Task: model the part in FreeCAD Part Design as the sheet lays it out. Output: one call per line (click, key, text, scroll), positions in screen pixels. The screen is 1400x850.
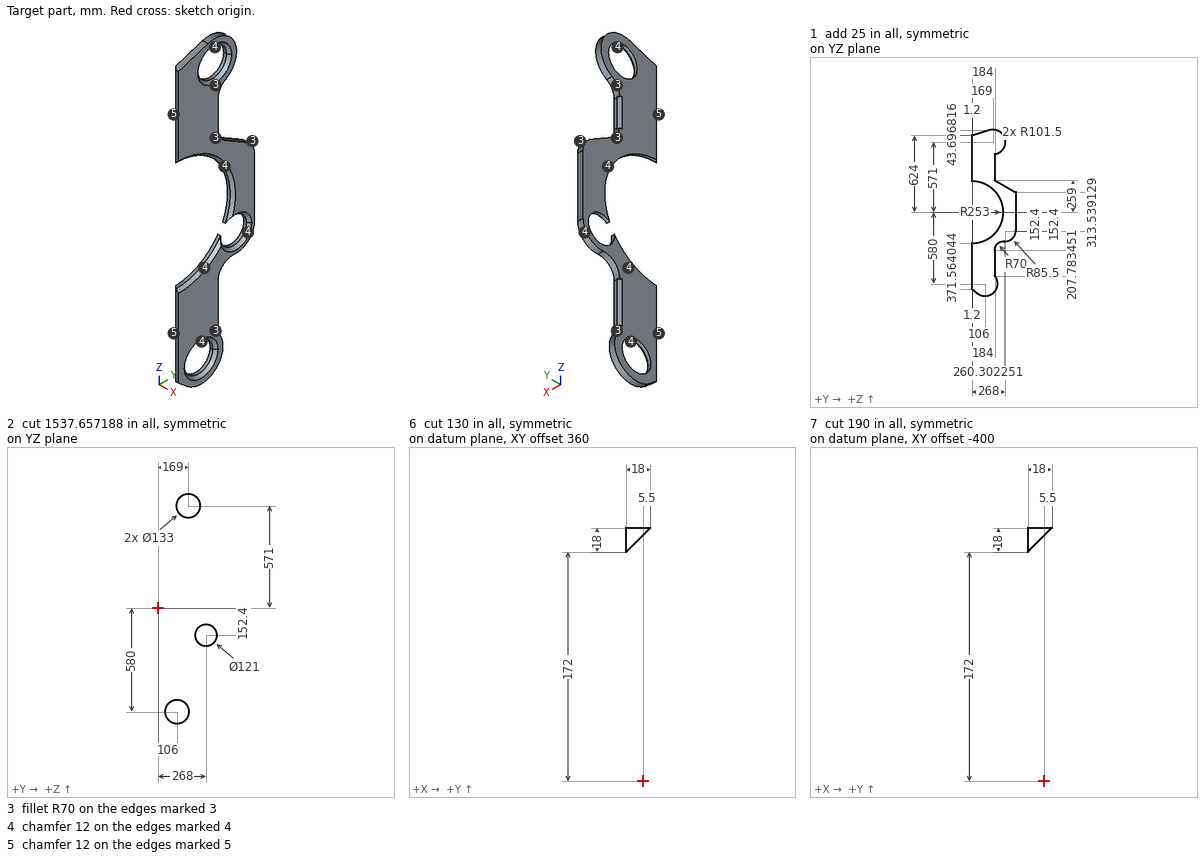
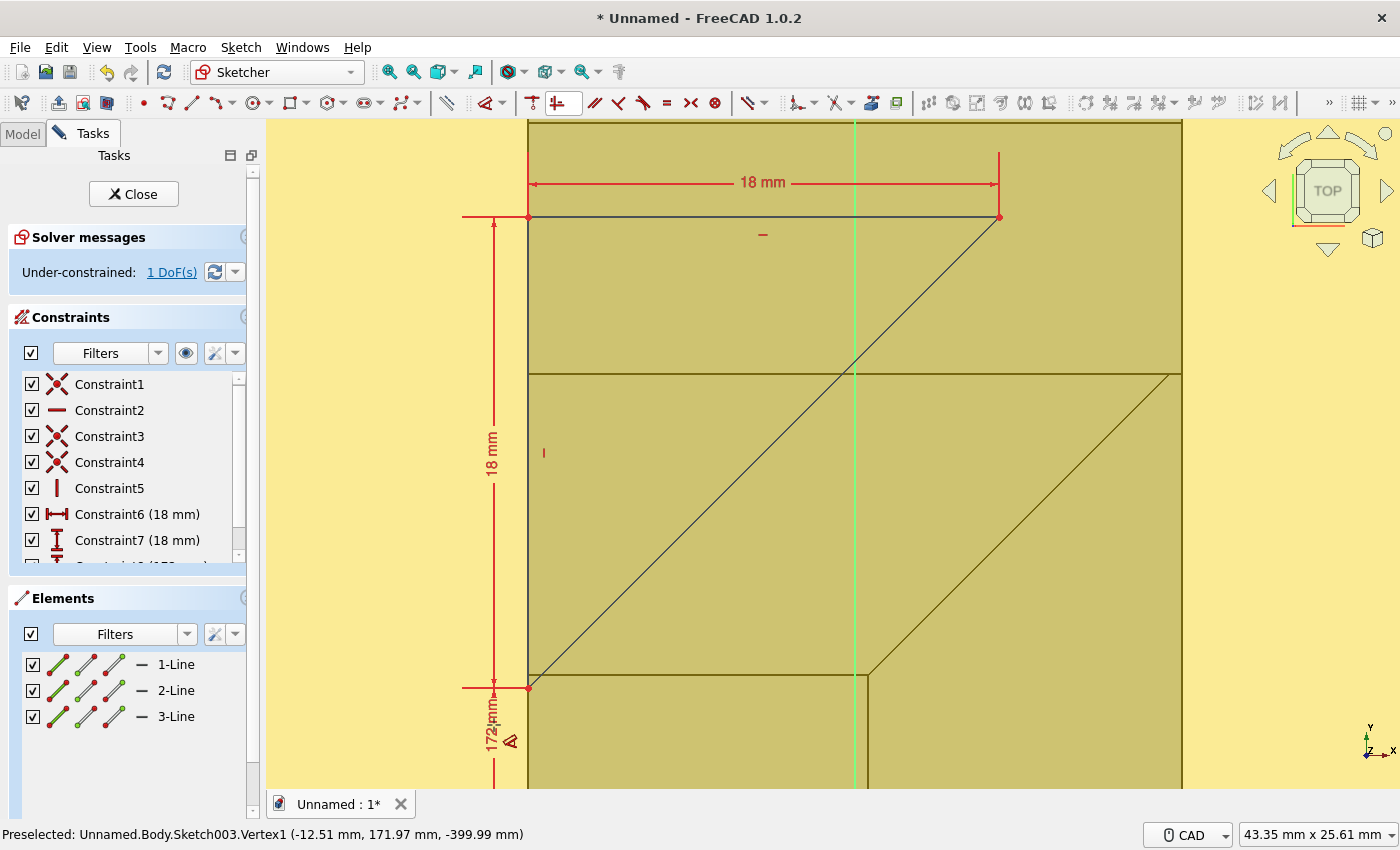
click(999, 217)
click(927, 183)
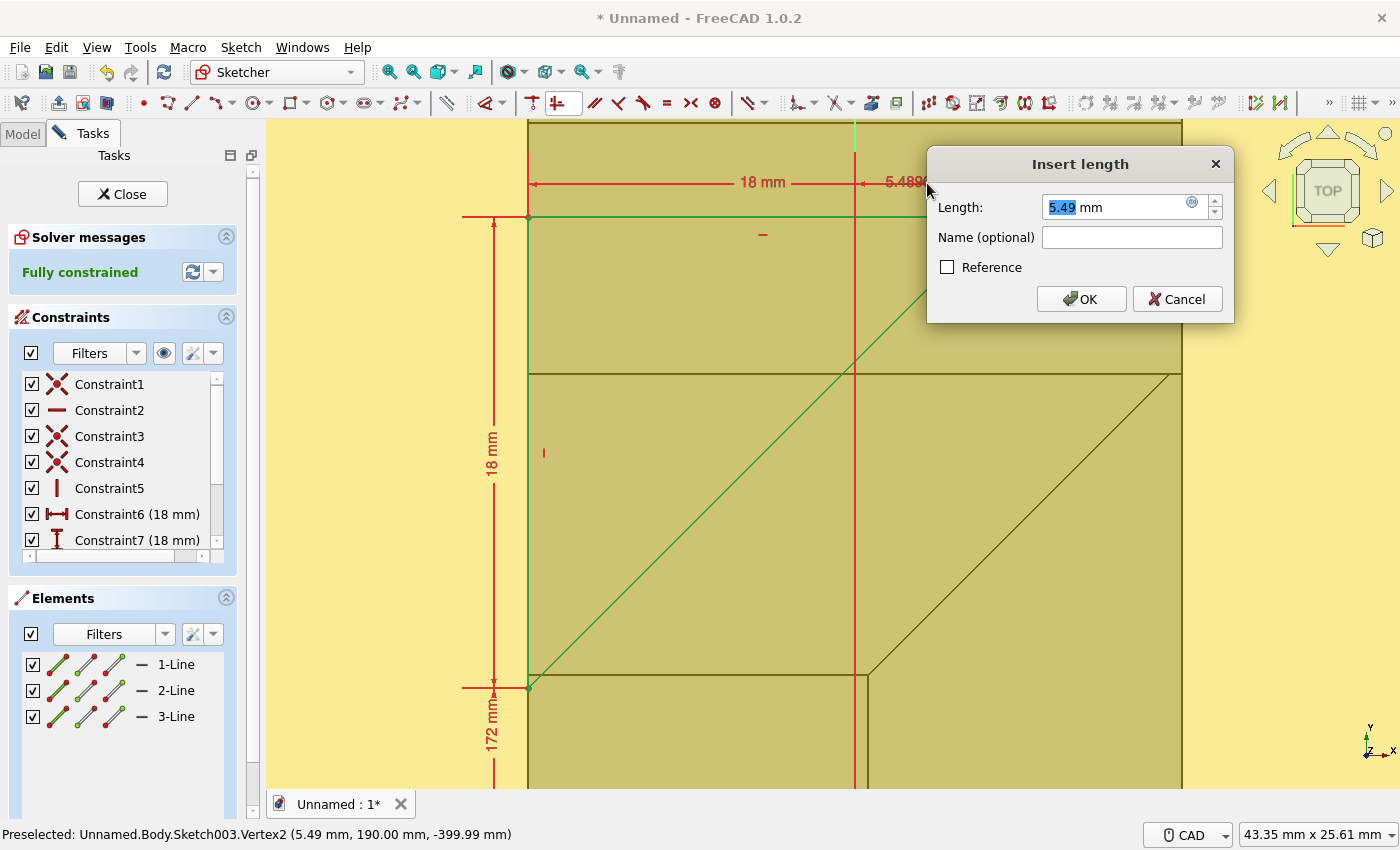
text(5.5)
key(Return)
key(Escape)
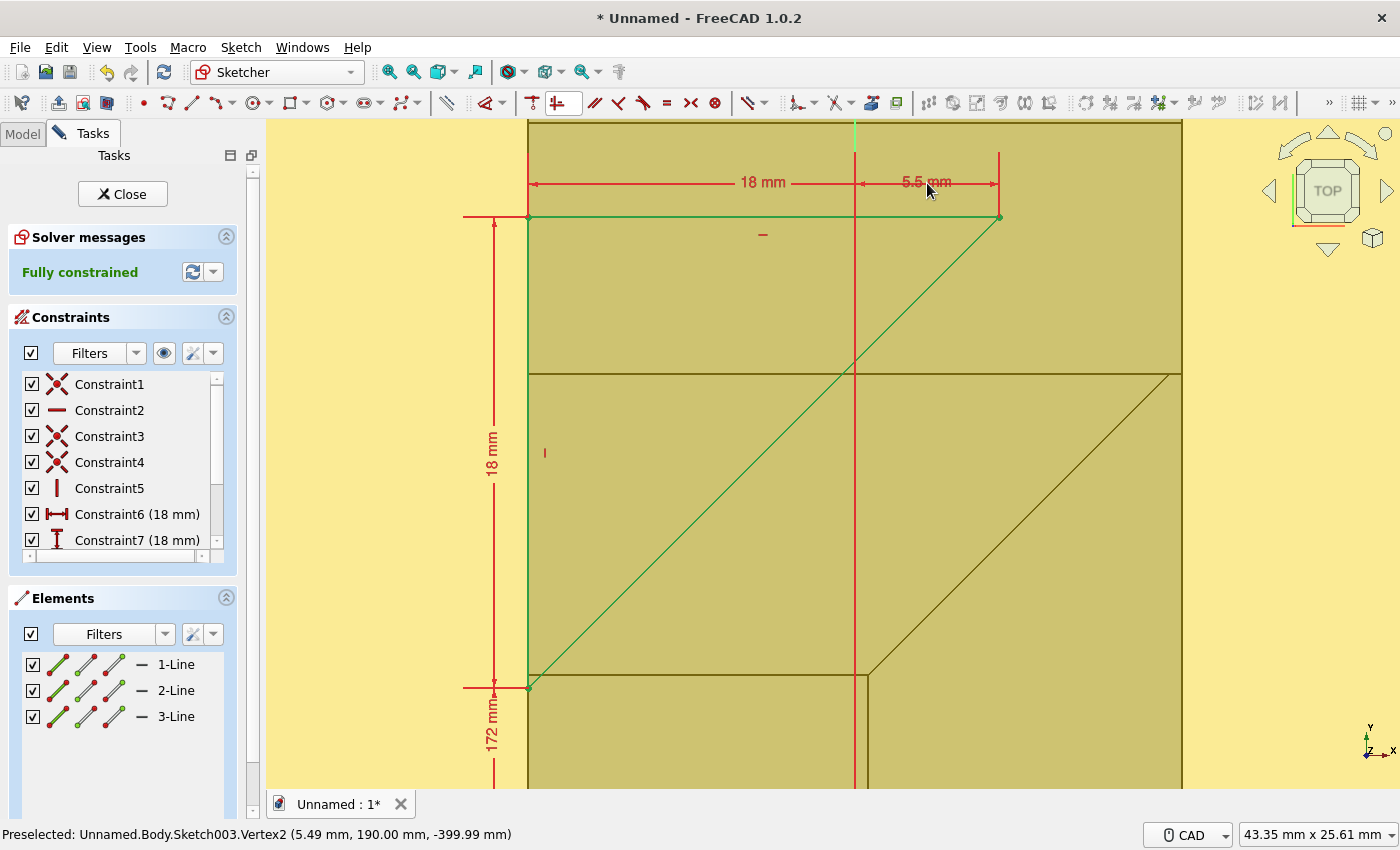
click(123, 194)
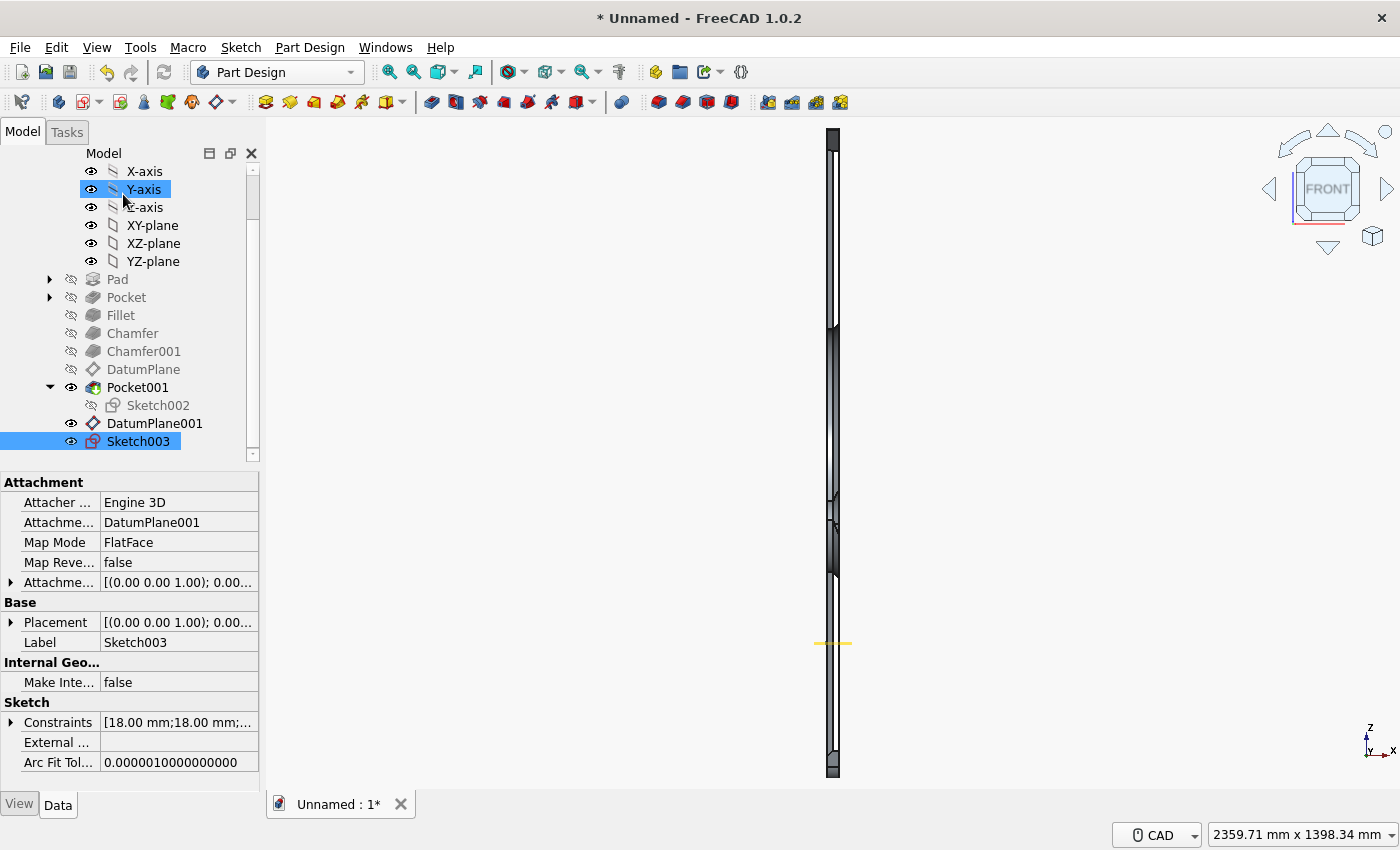
click(432, 102)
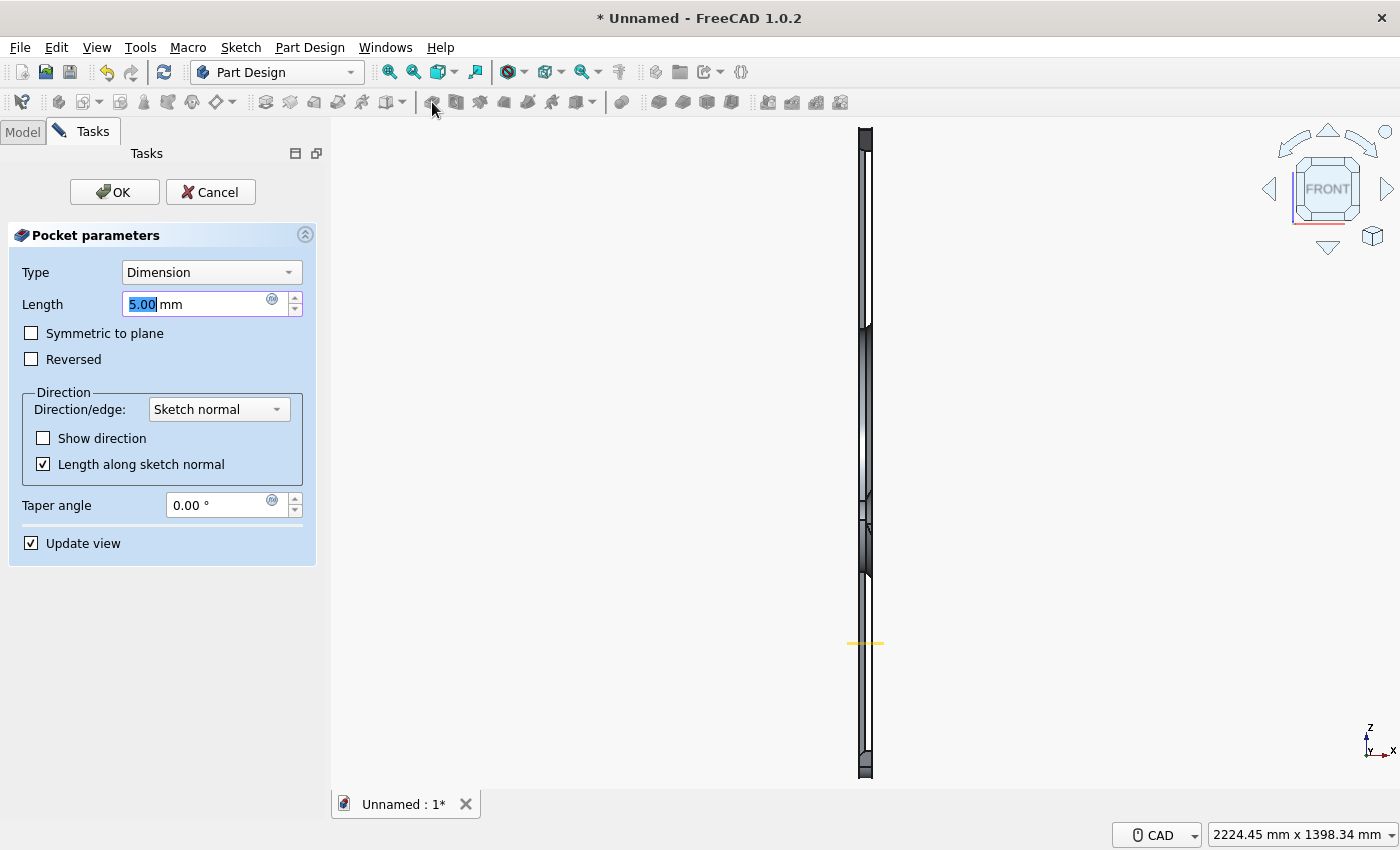
text(190)
key(Tab)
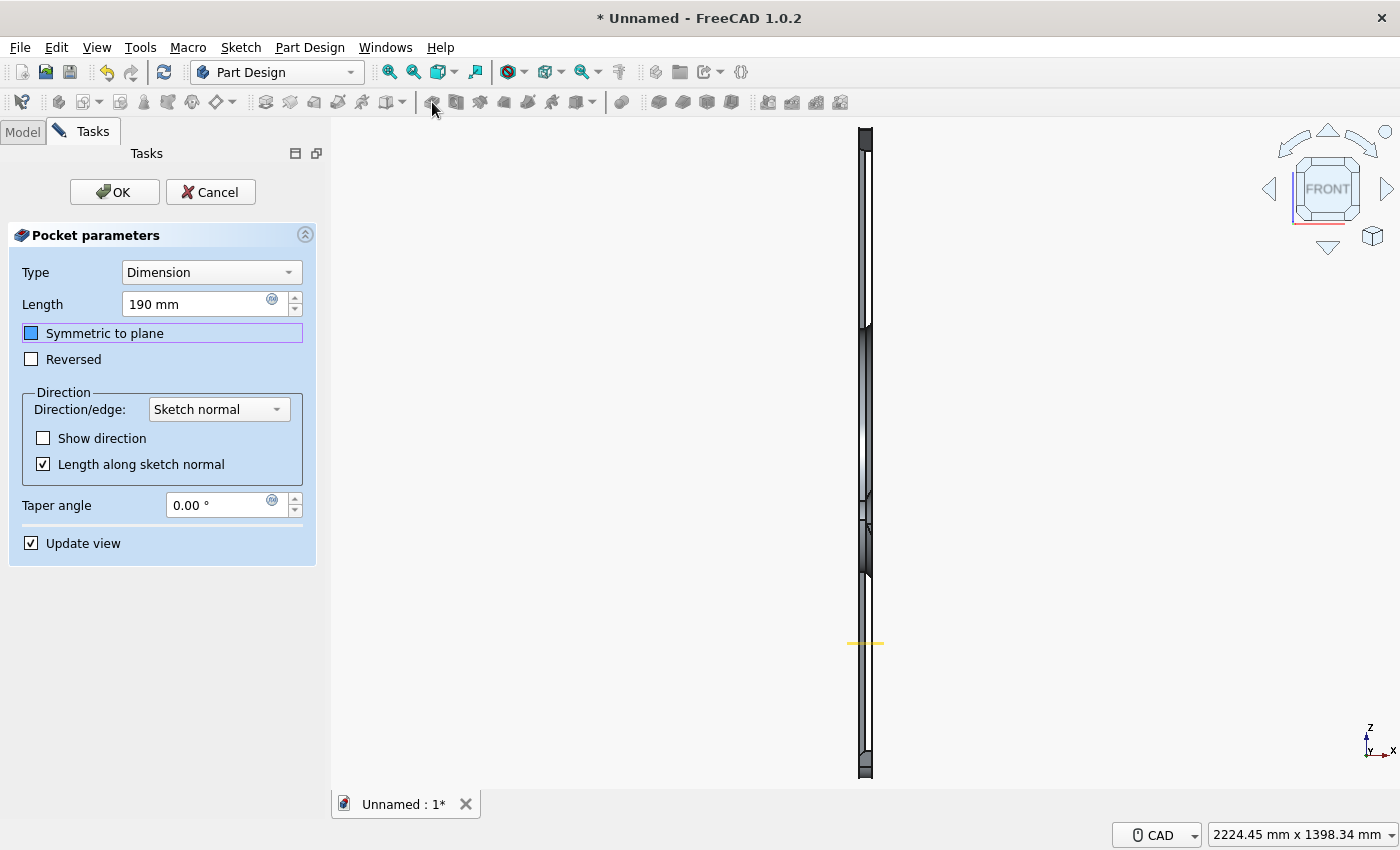
click(30, 333)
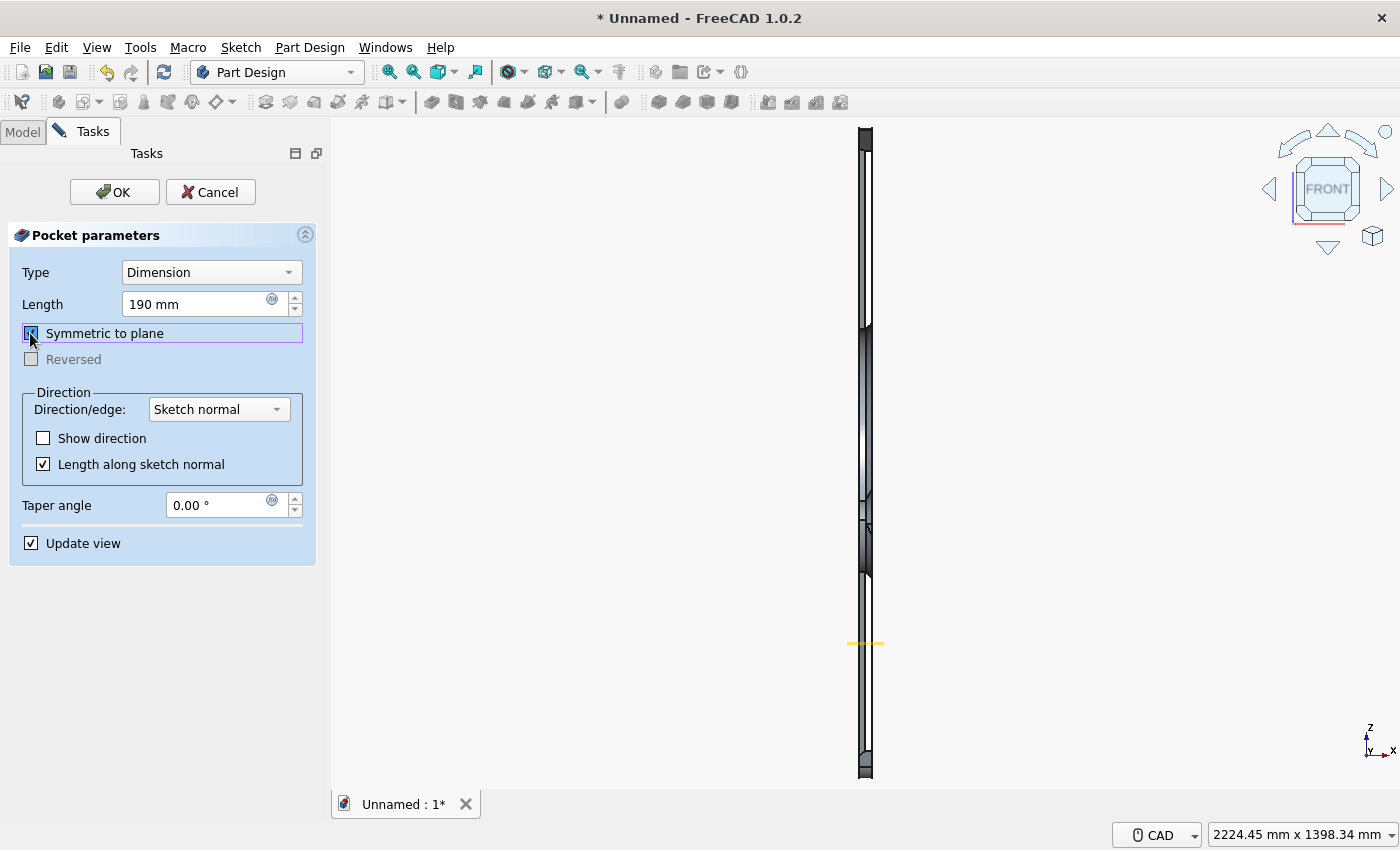
click(115, 192)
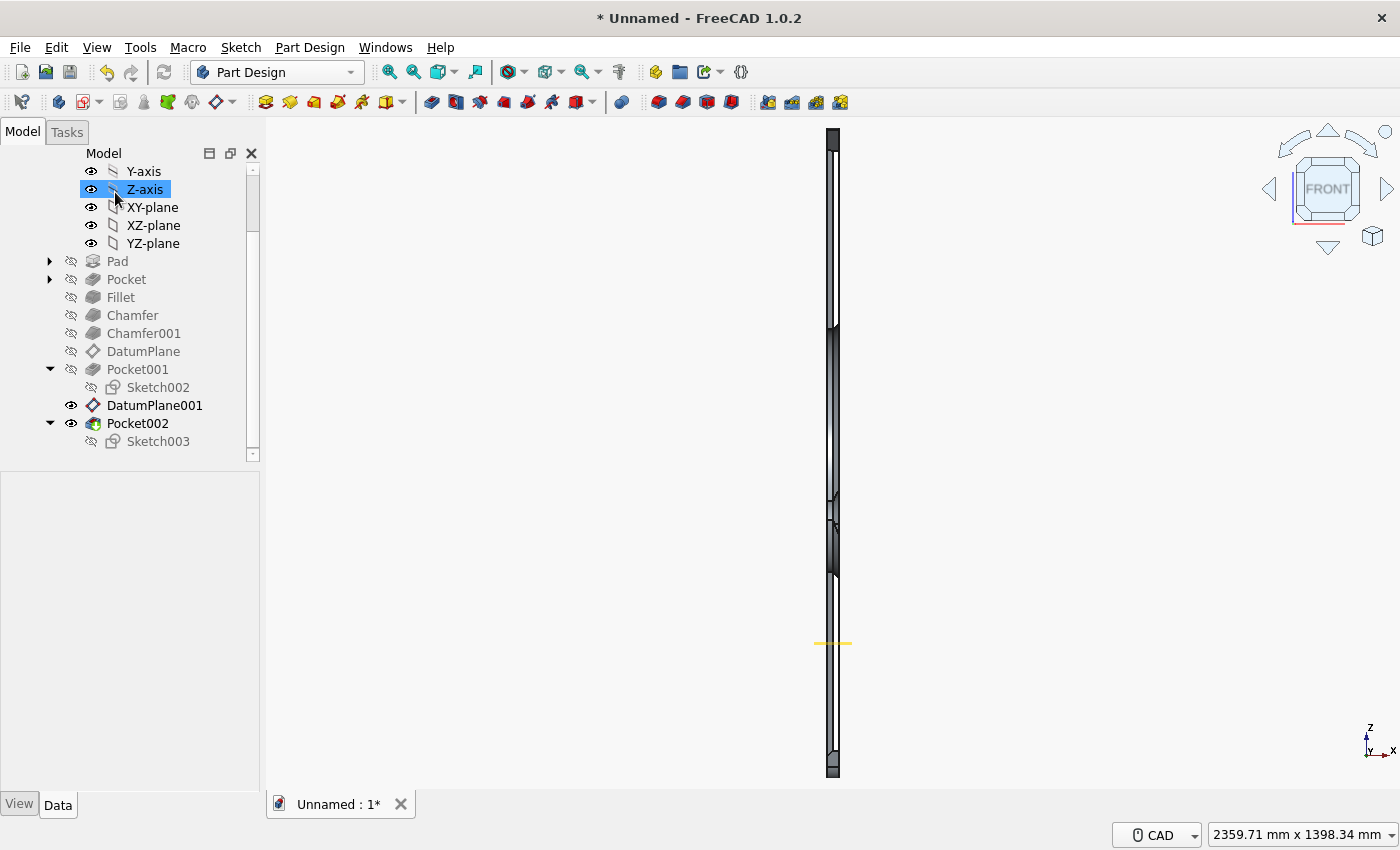
click(116, 405)
key(space)